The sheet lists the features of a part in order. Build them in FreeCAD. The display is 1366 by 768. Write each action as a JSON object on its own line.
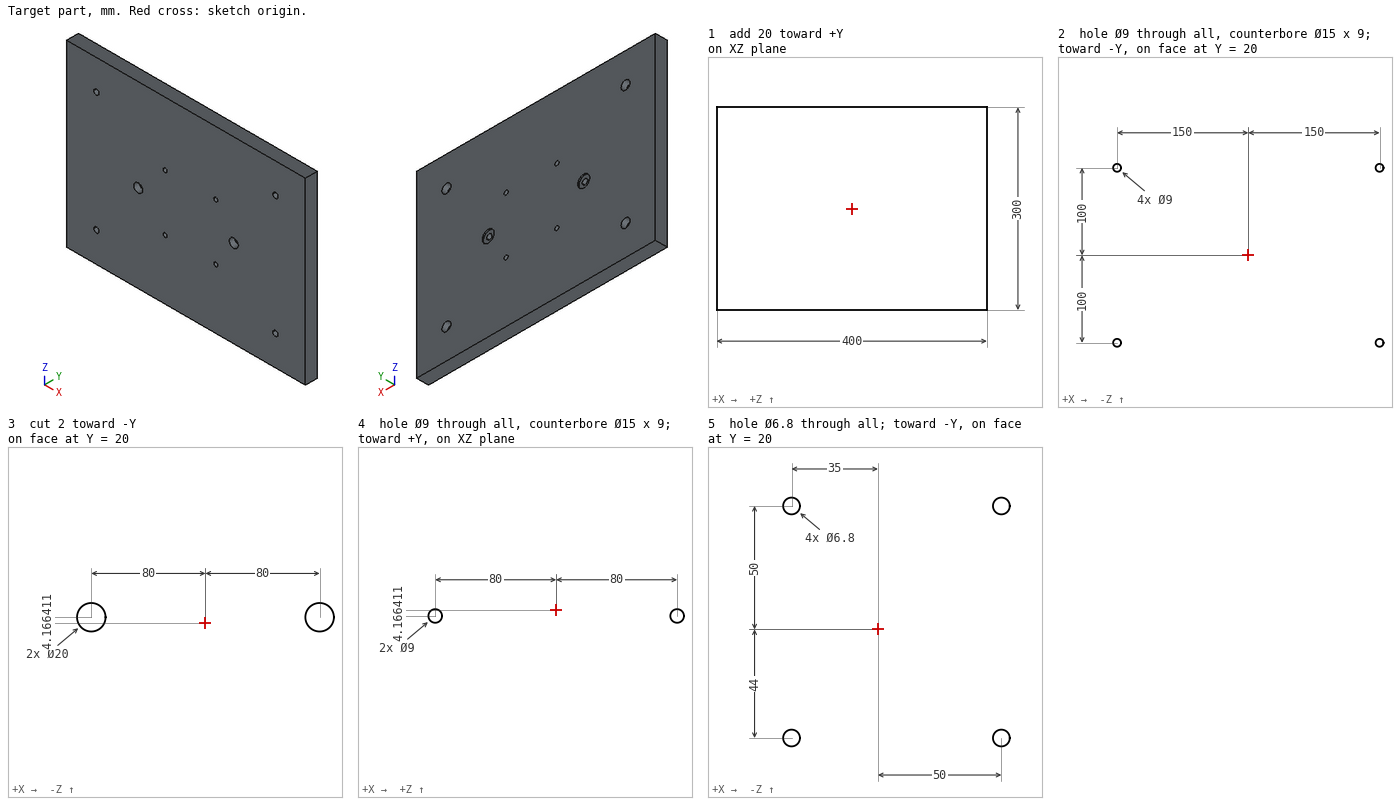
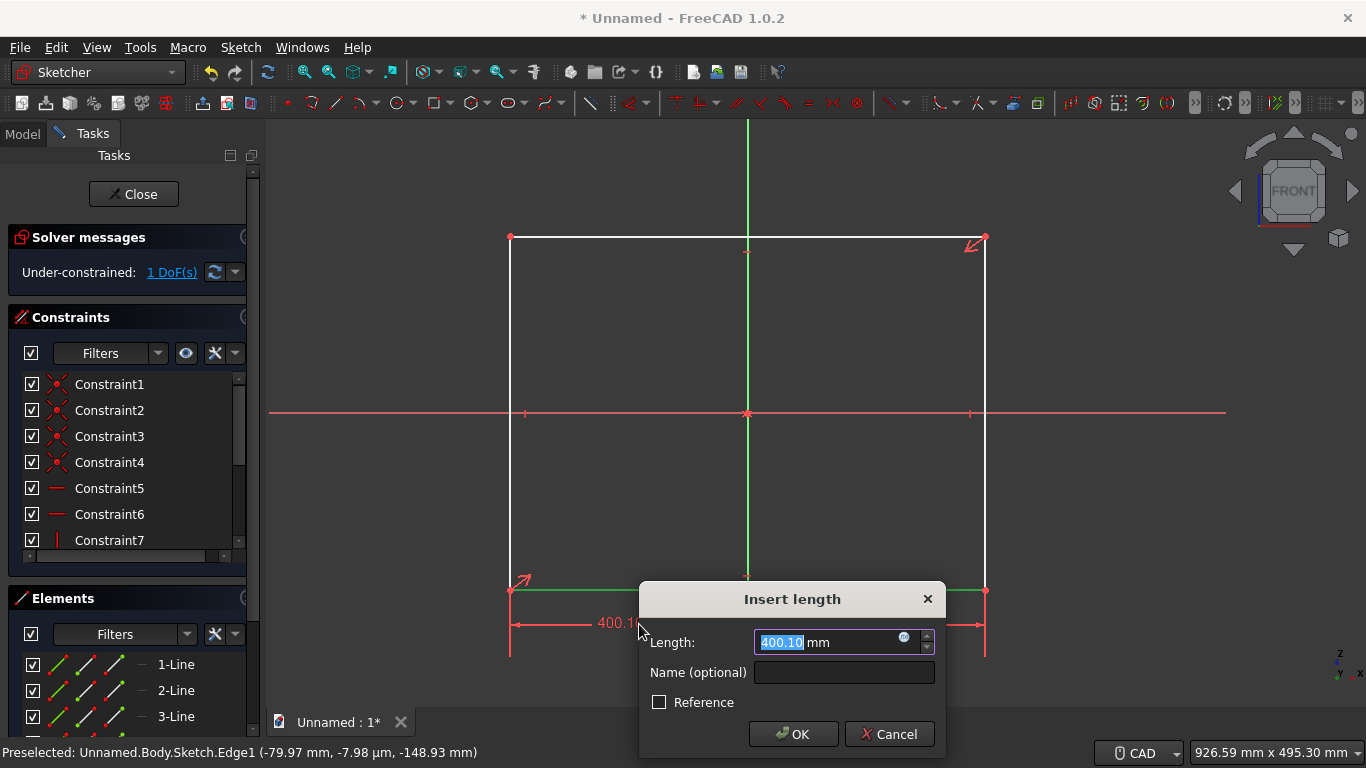
{"action": "type", "text": "400"}
{"action": "key", "text": "Return"}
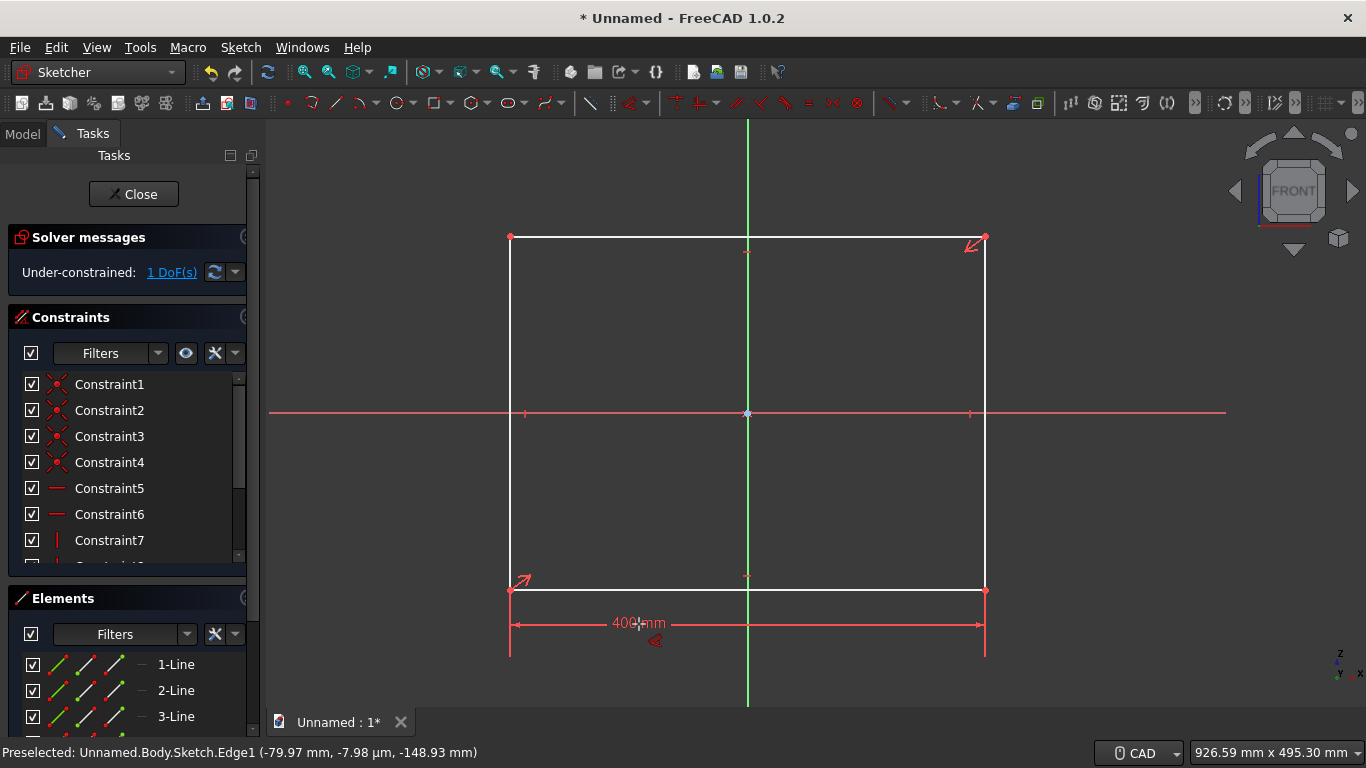
{"action": "left_click", "coordinate": [985, 484]}
{"action": "left_click", "coordinate": [1019, 332]}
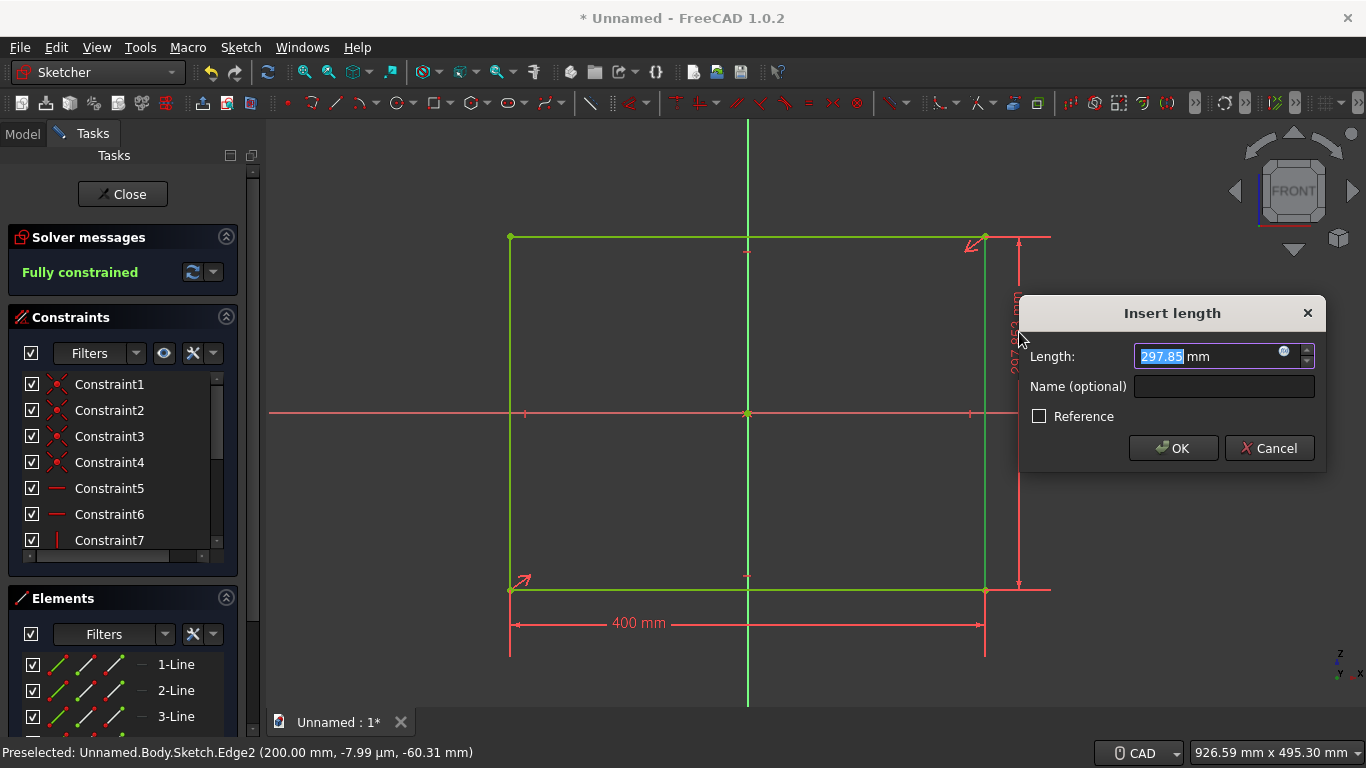
{"action": "type", "text": "300"}
{"action": "key", "text": "Return"}
{"action": "key", "text": "Escape"}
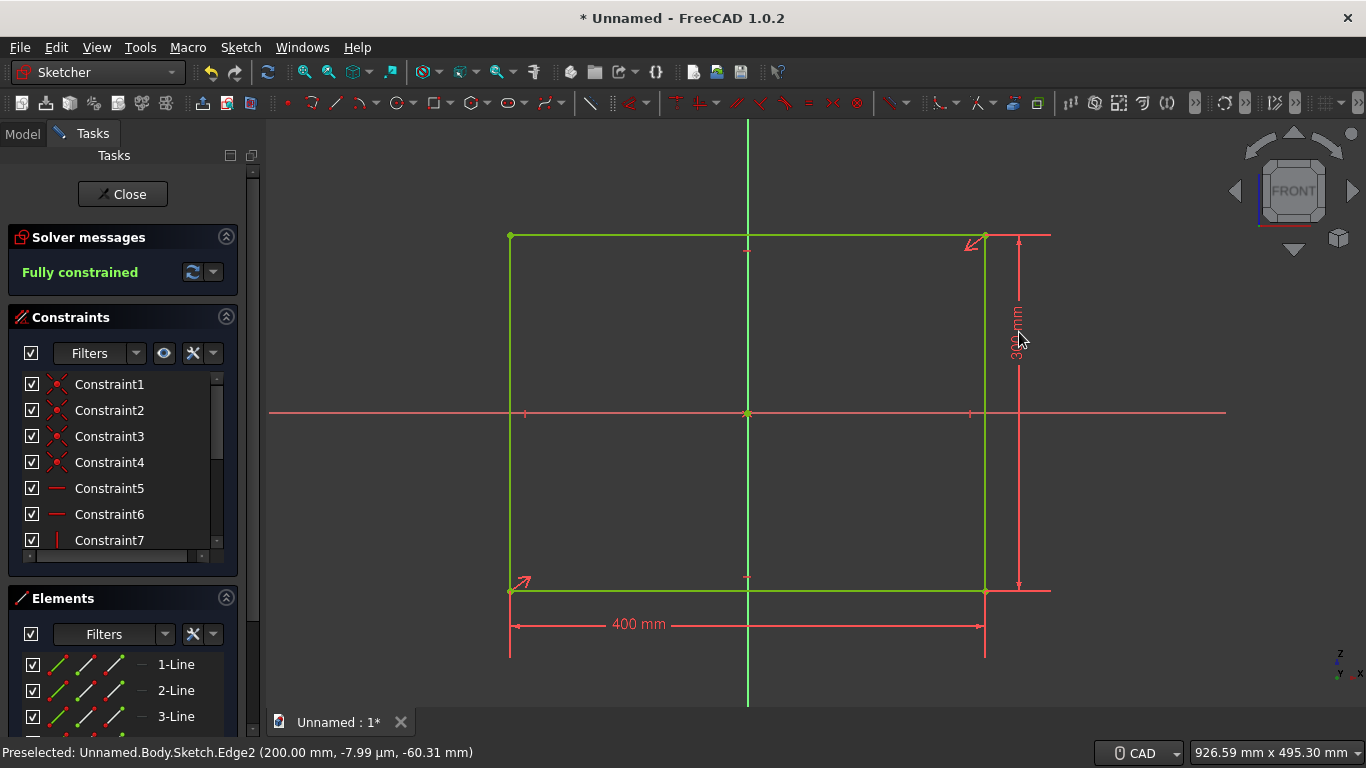
{"action": "left_click", "coordinate": [123, 194]}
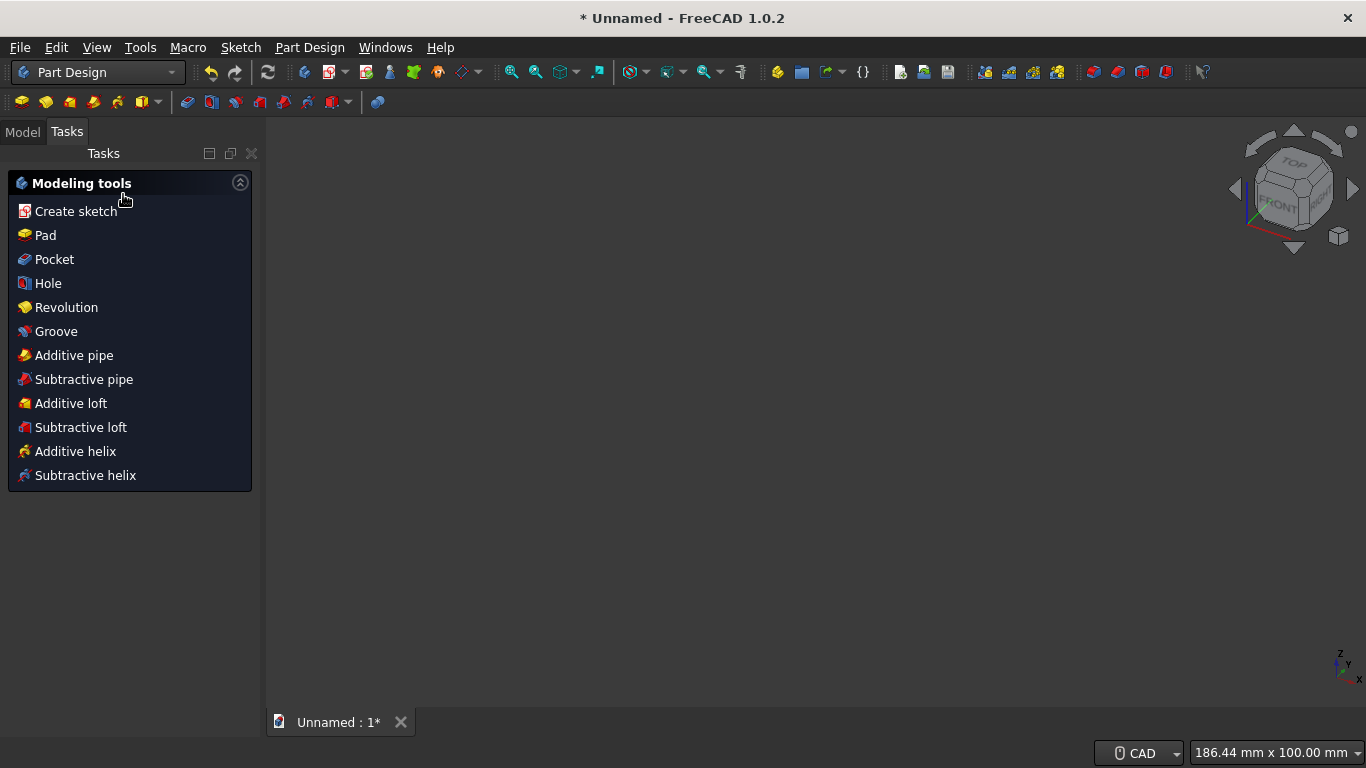
{"action": "left_click", "coordinate": [22, 102]}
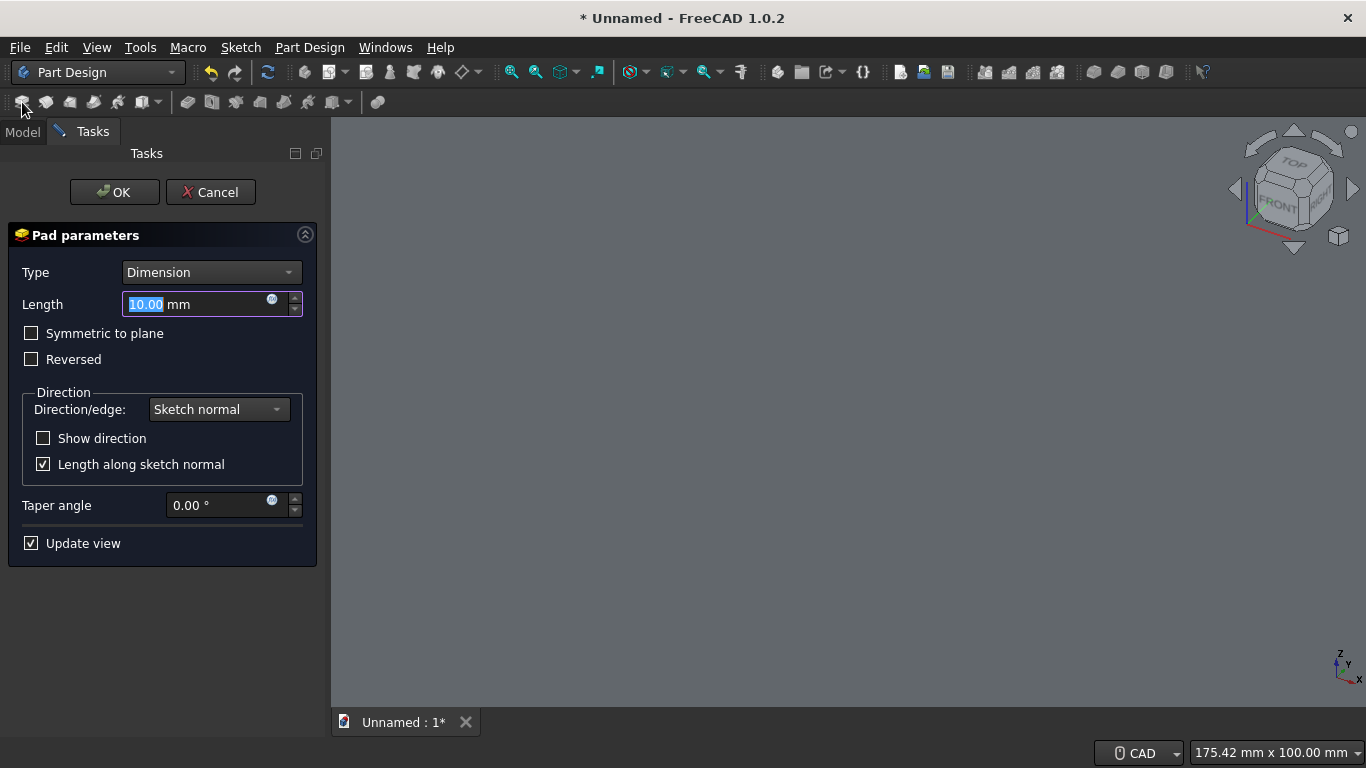
{"action": "type", "text": "20"}
{"action": "key", "text": "Tab"}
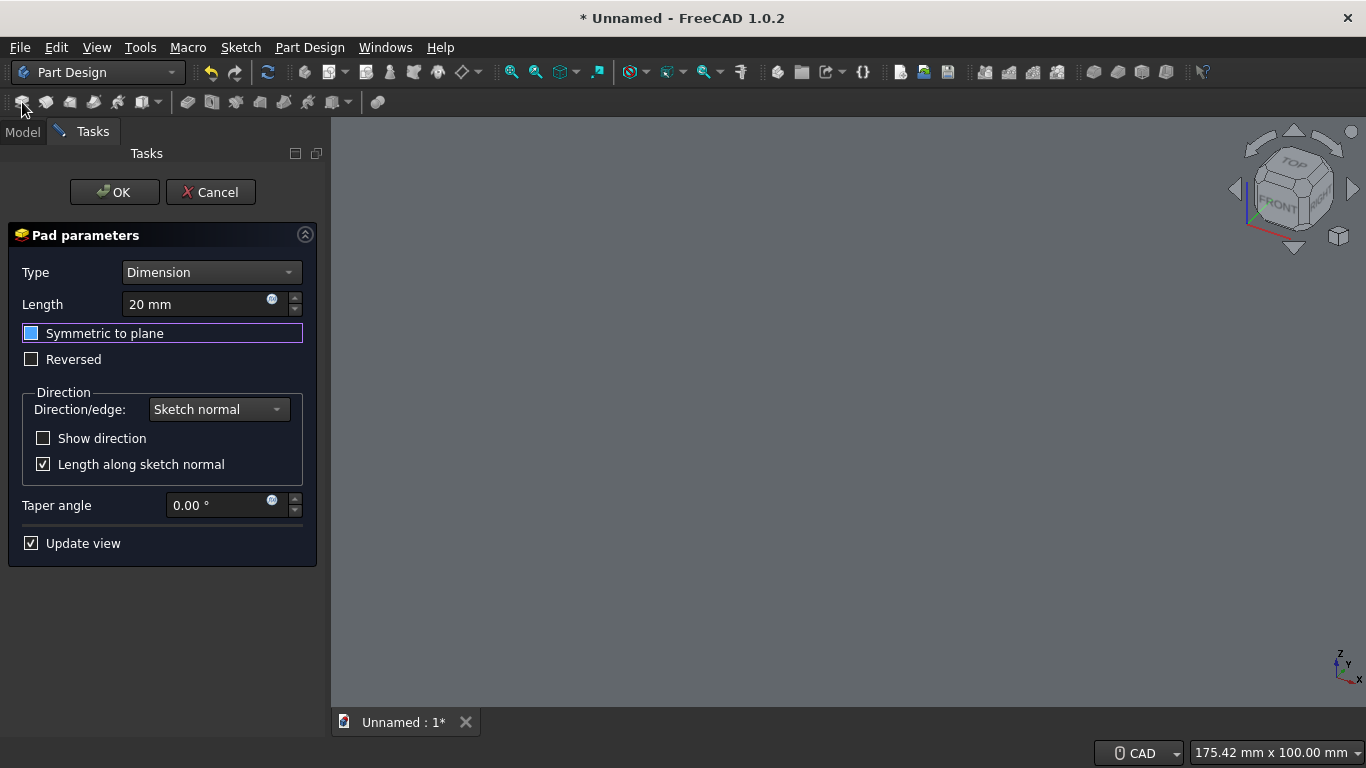
{"action": "left_click", "coordinate": [30, 359]}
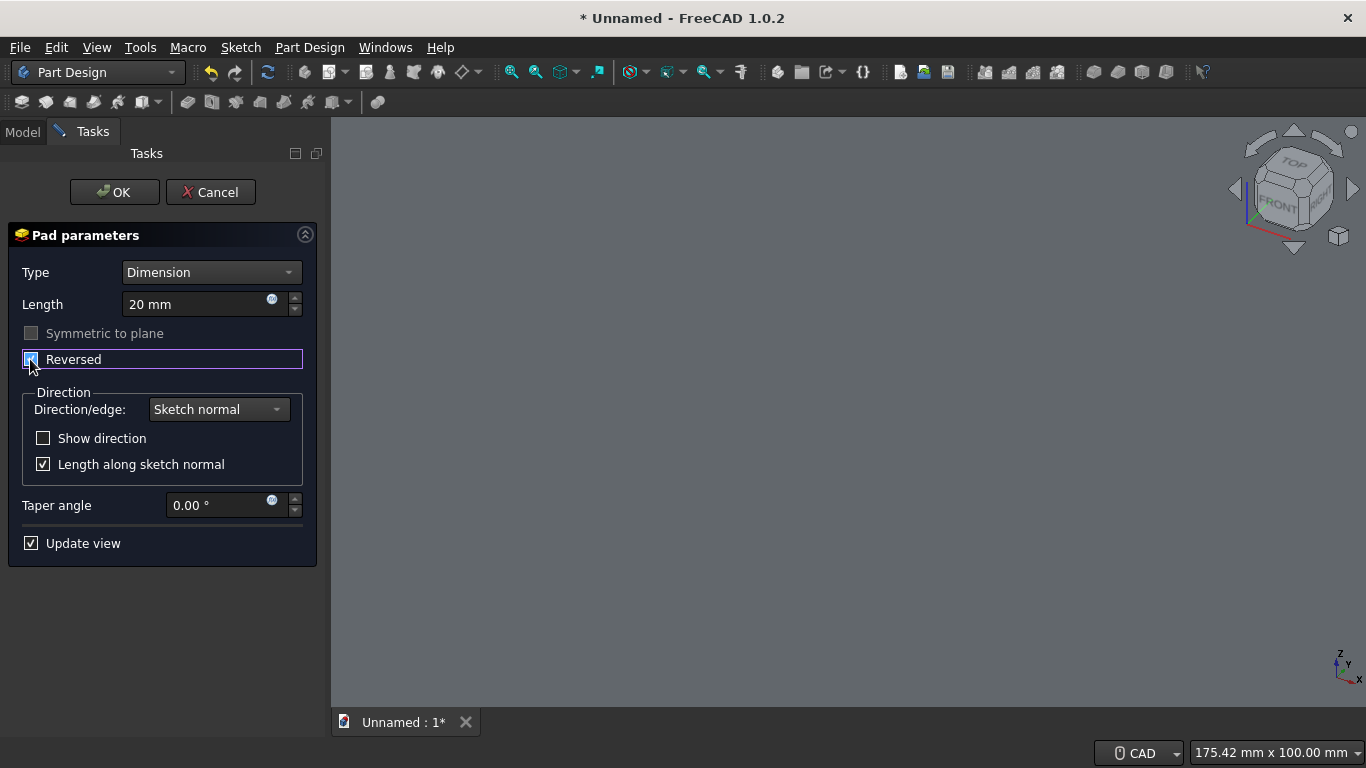
{"action": "left_click", "coordinate": [115, 192]}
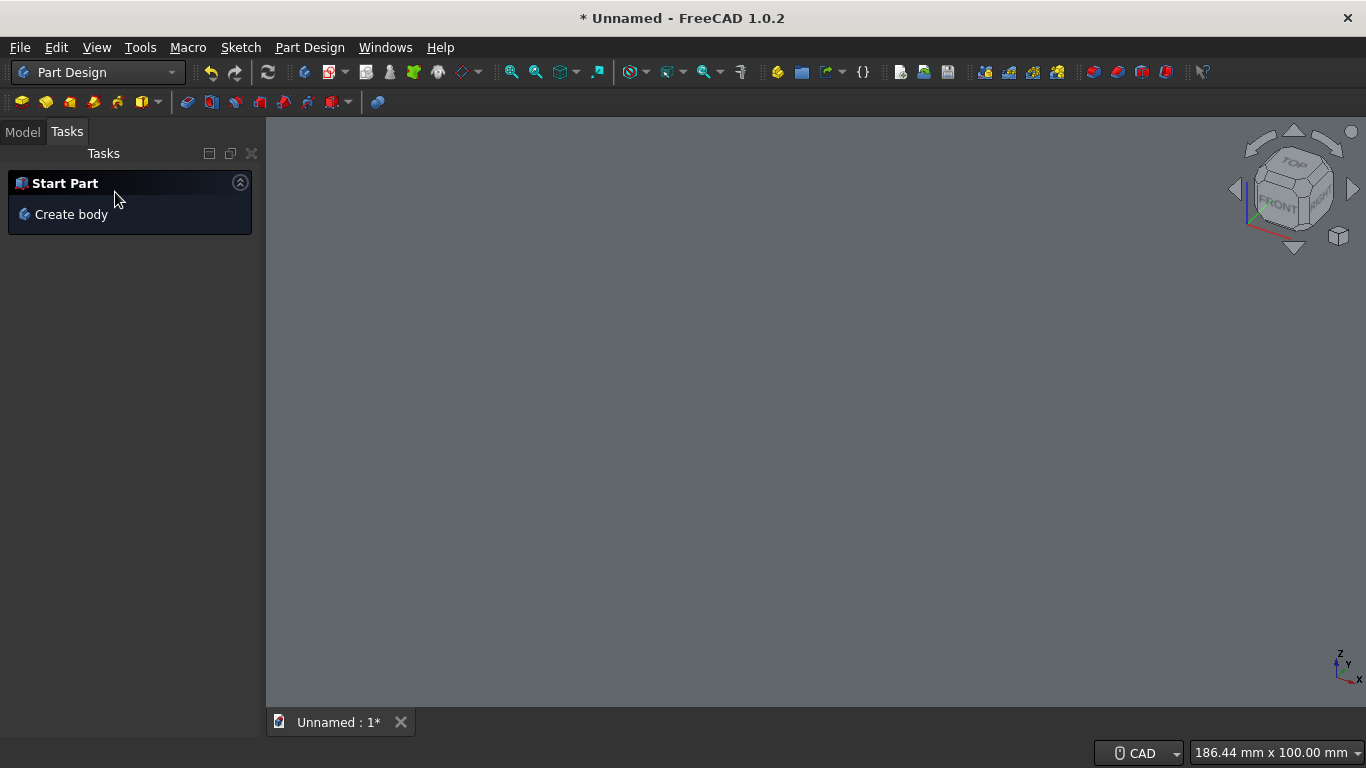
{"action": "left_click", "coordinate": [512, 72]}